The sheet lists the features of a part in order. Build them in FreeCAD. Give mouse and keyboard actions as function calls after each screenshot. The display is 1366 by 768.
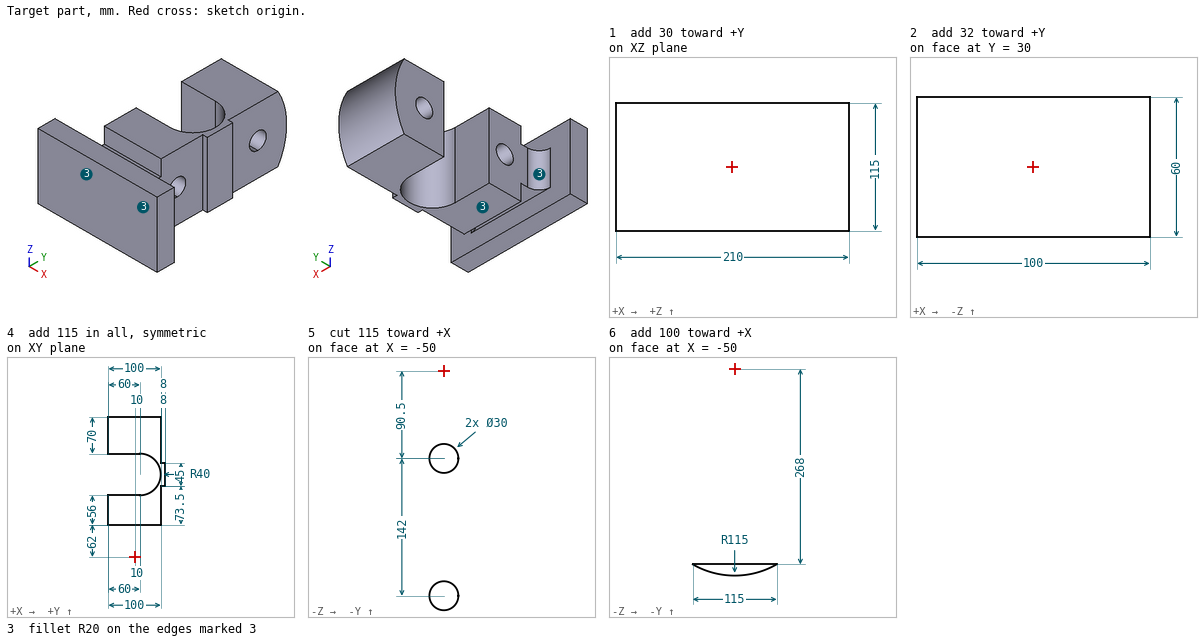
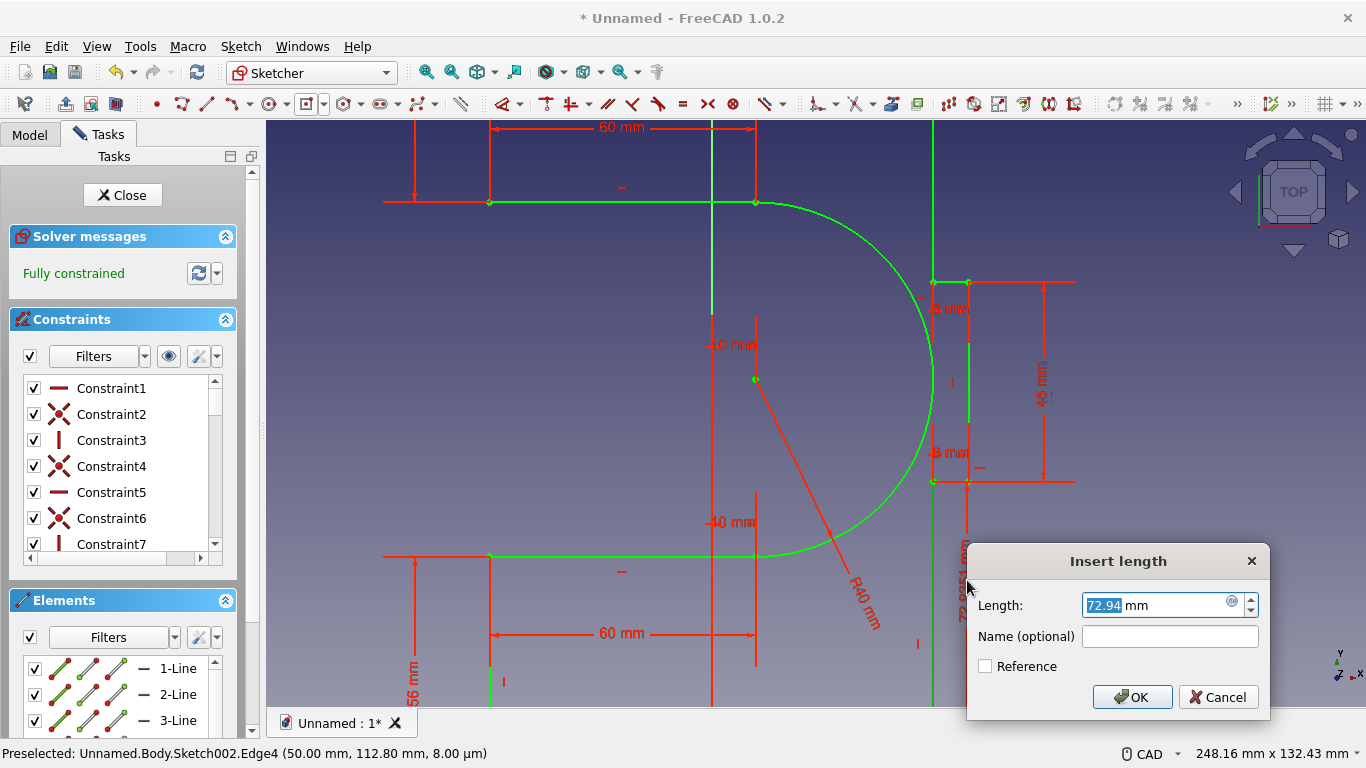
text(73.5)
key(Return)
key(Escape)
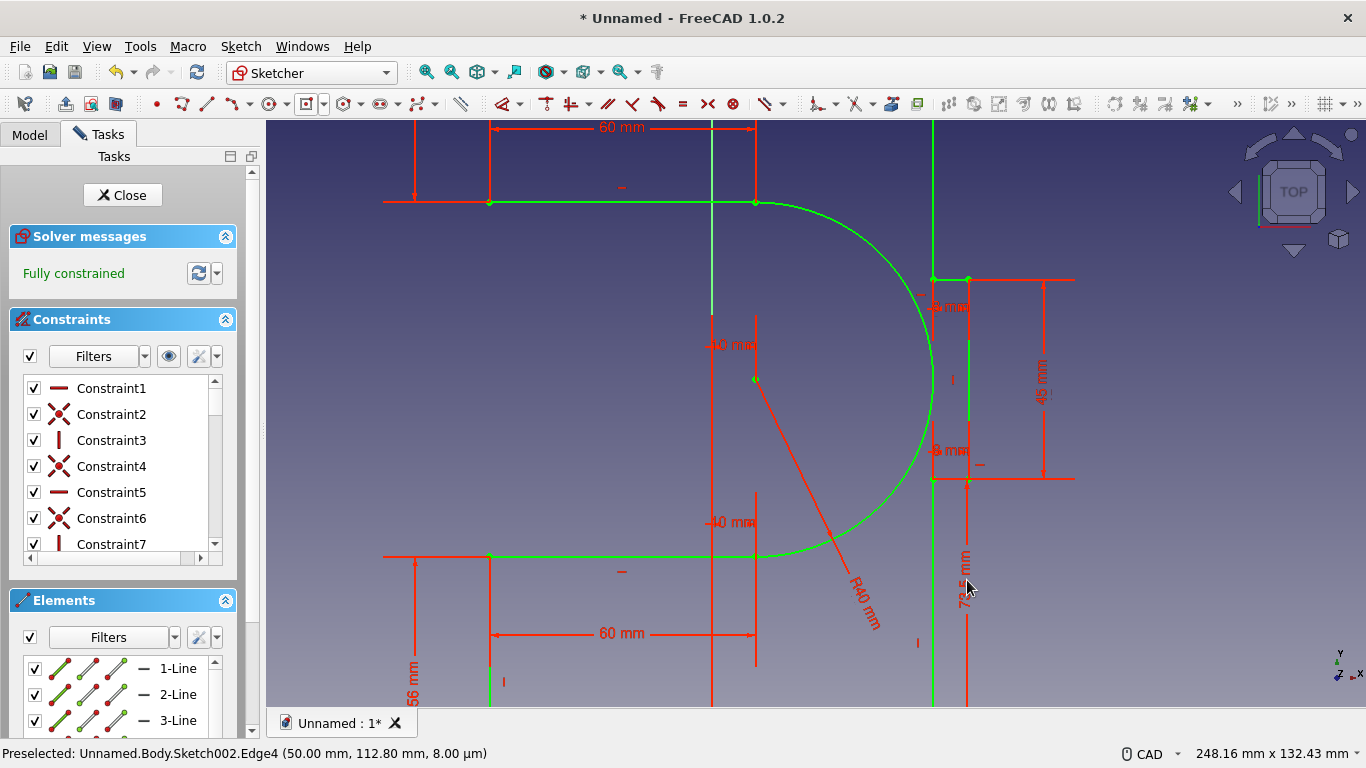
click(123, 195)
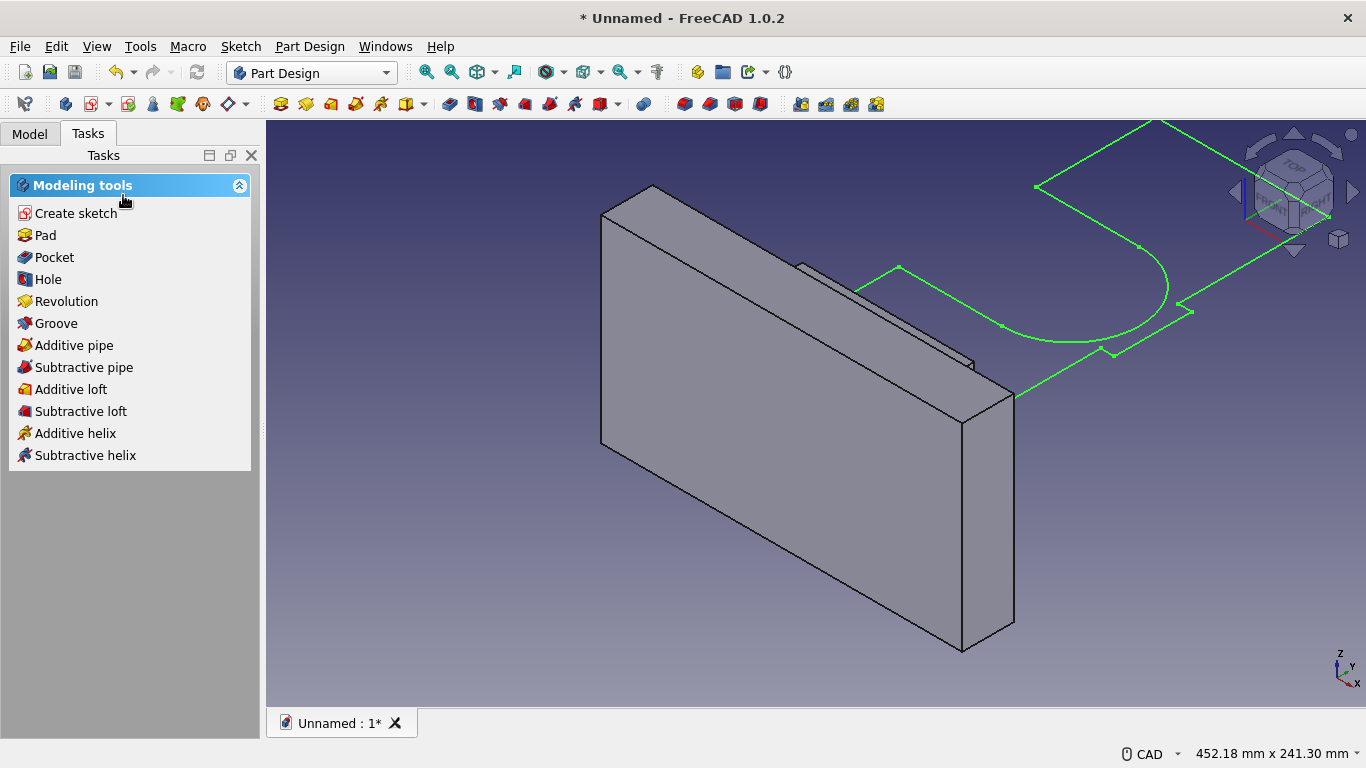
click(281, 104)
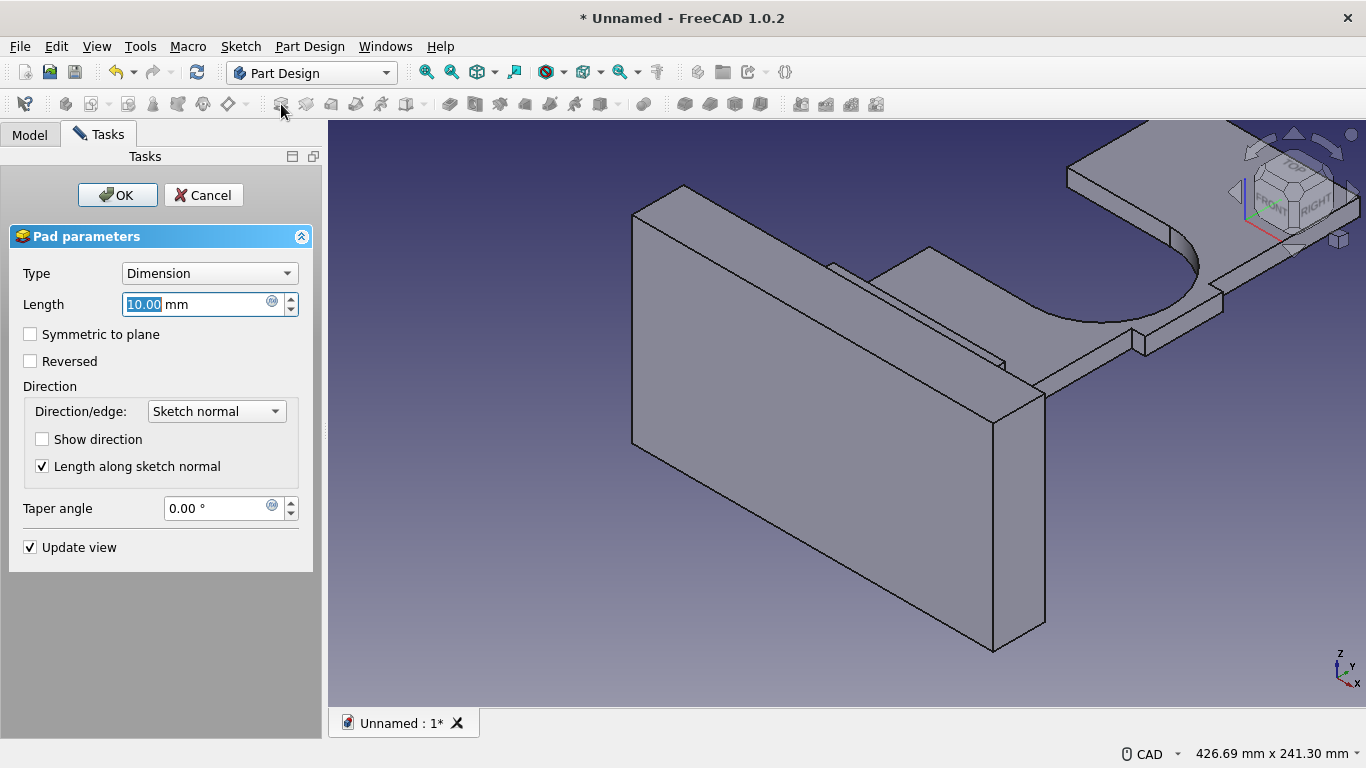
text(115)
key(Tab)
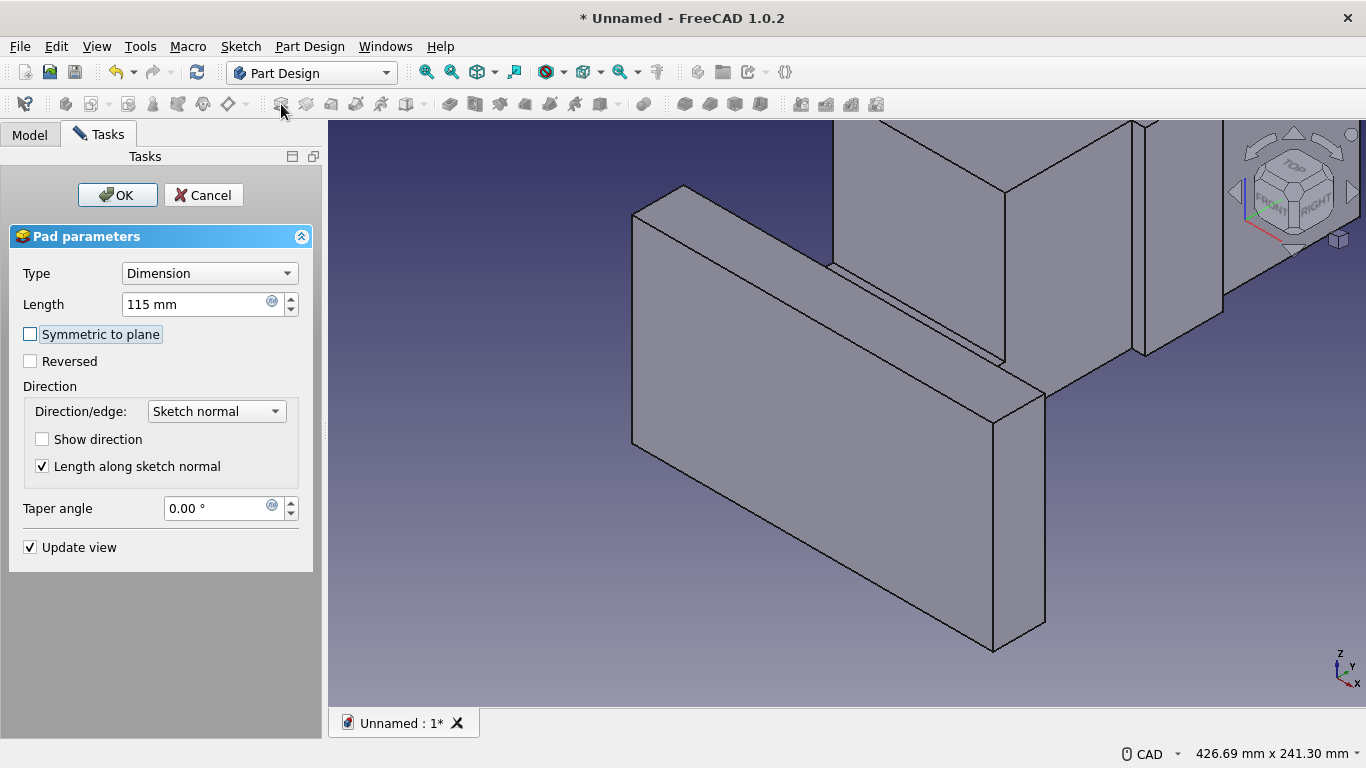
click(31, 334)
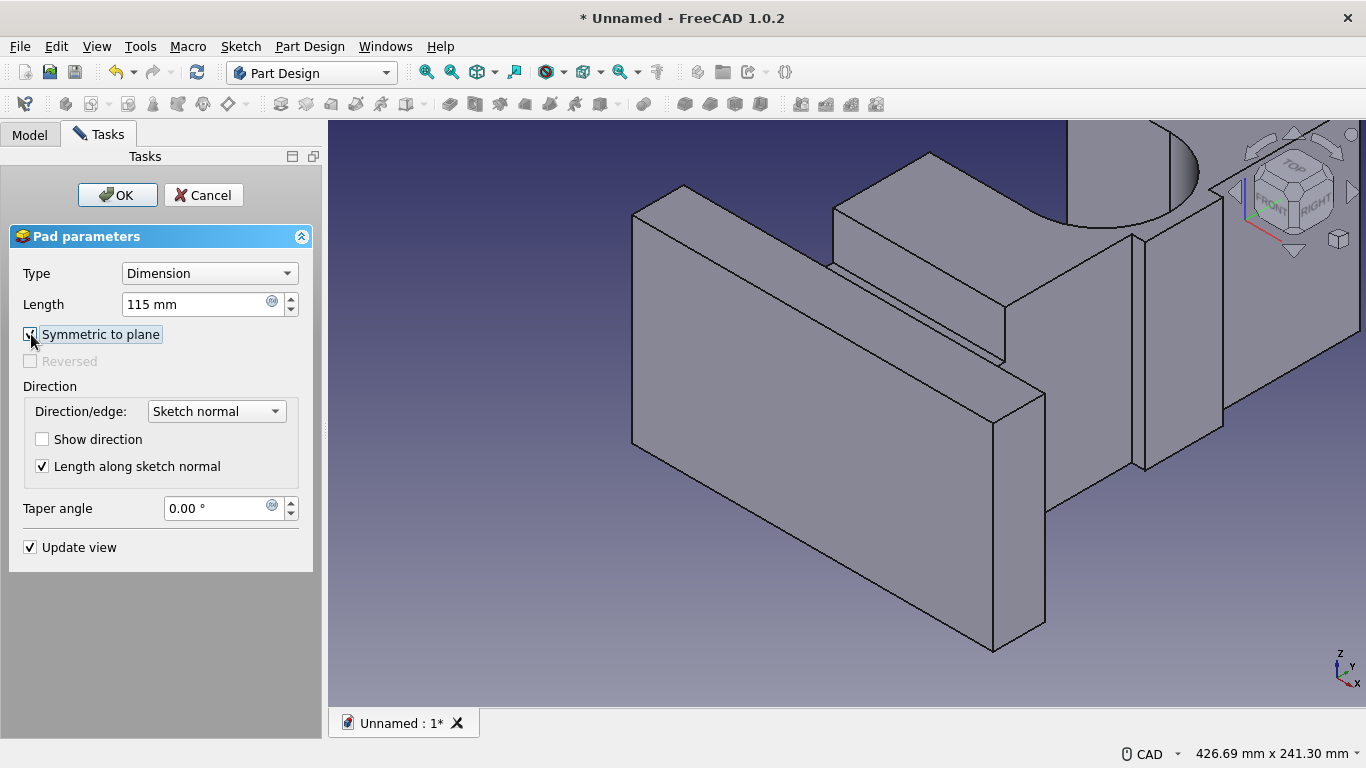
click(118, 195)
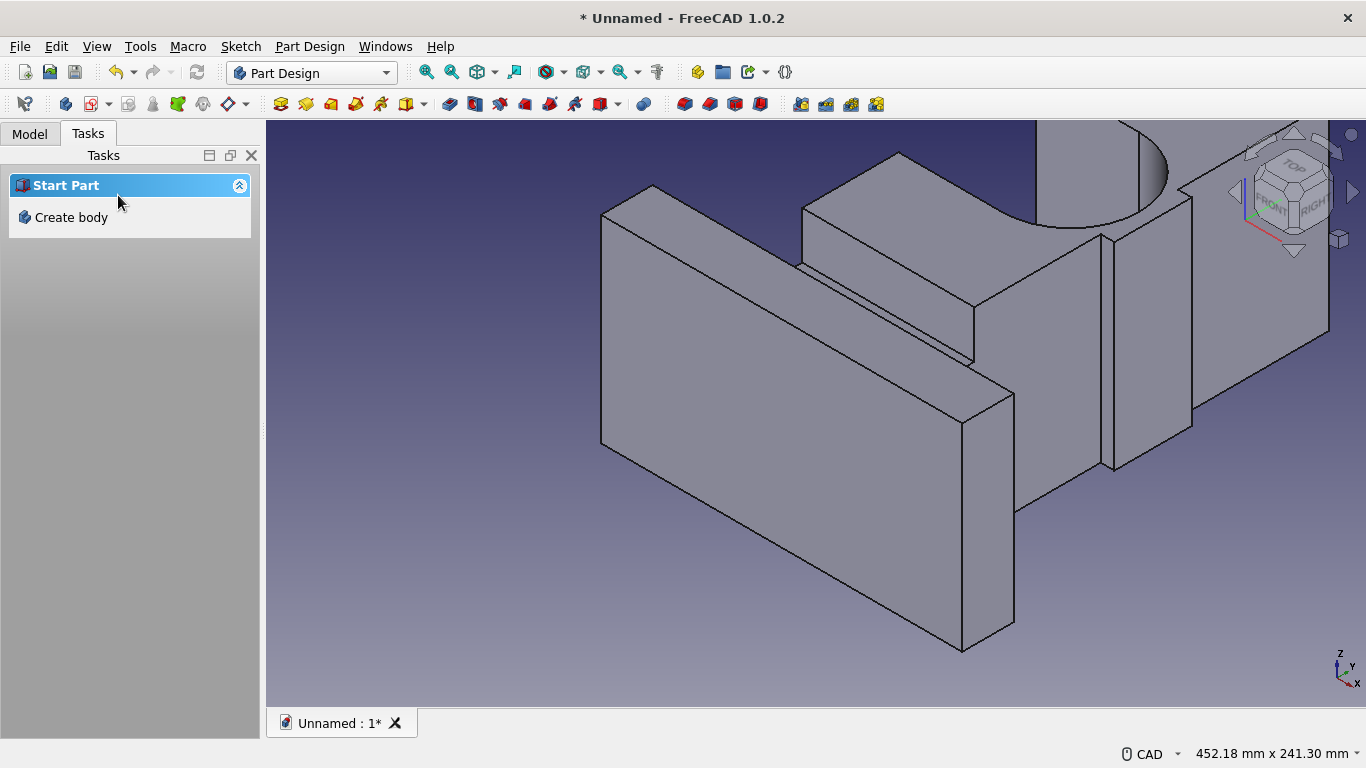
click(427, 72)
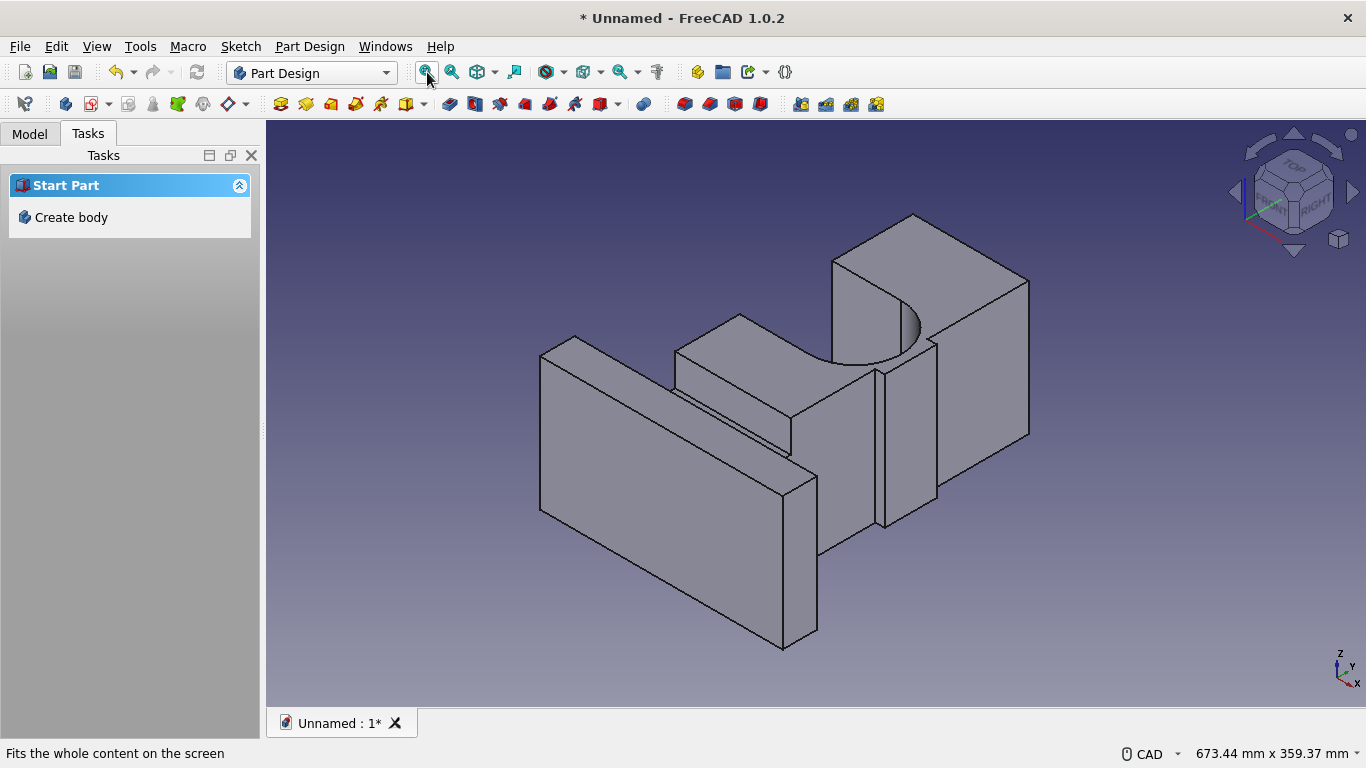
key(6)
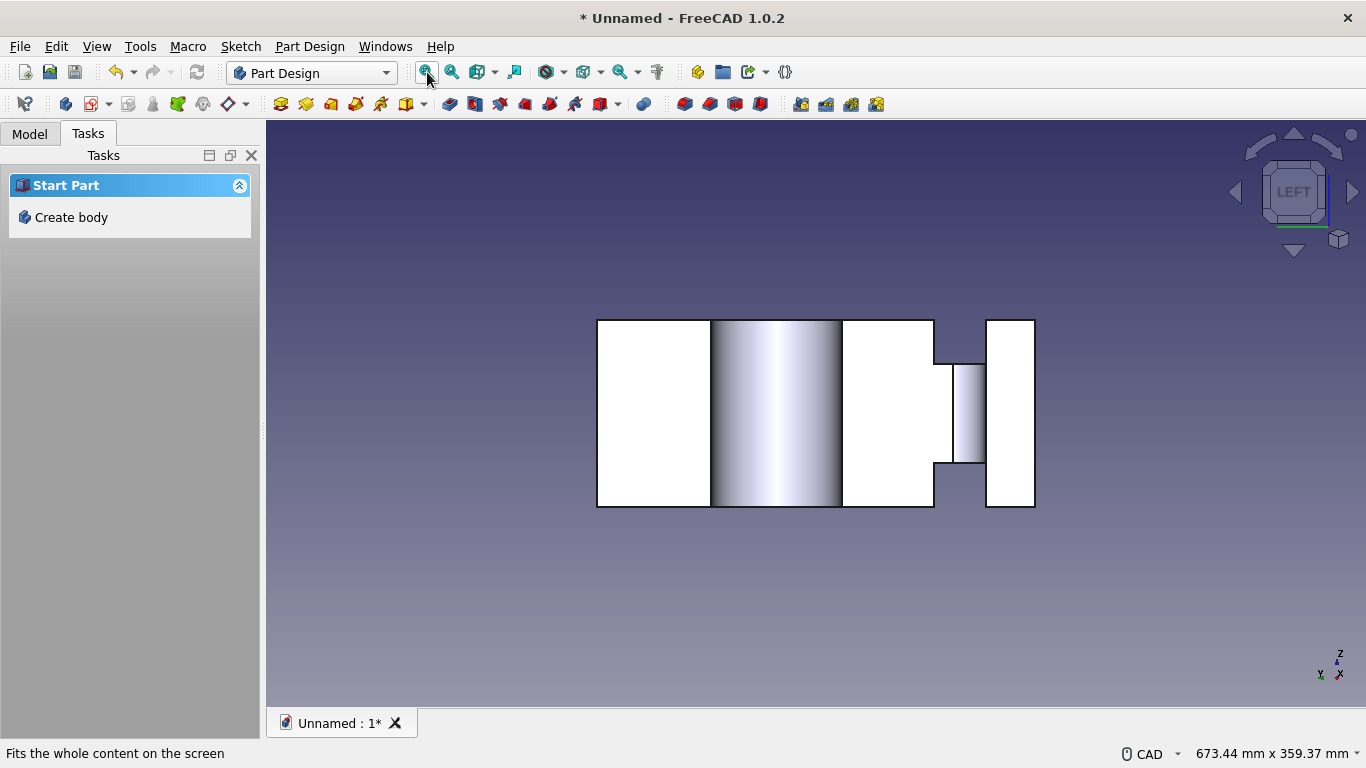
key(v)
key(f)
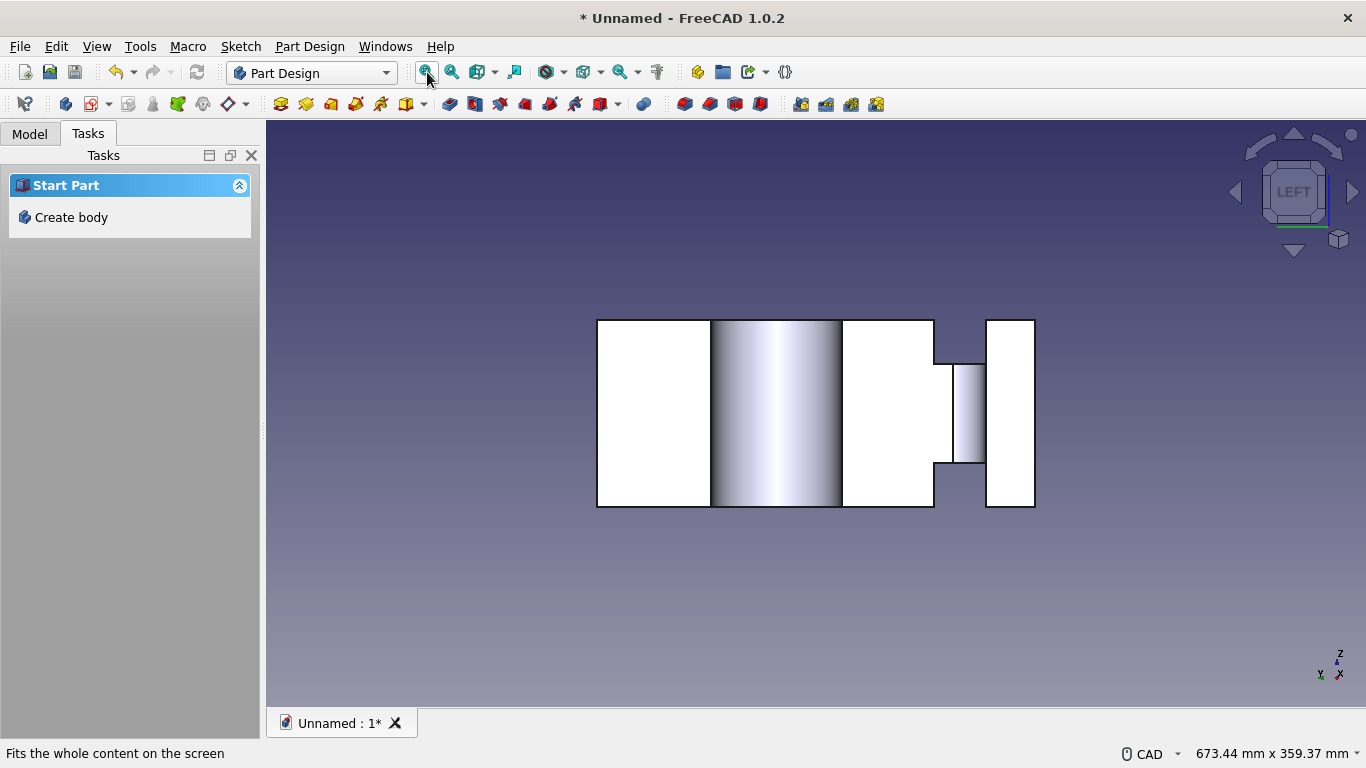
click(654, 386)